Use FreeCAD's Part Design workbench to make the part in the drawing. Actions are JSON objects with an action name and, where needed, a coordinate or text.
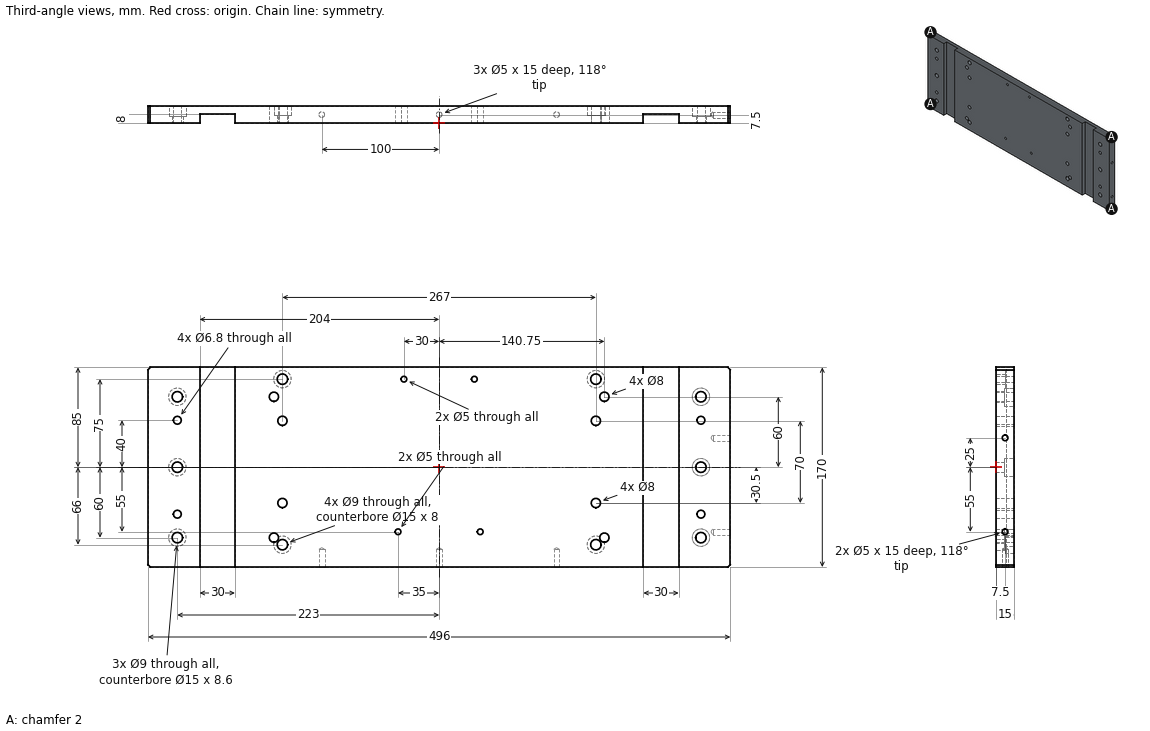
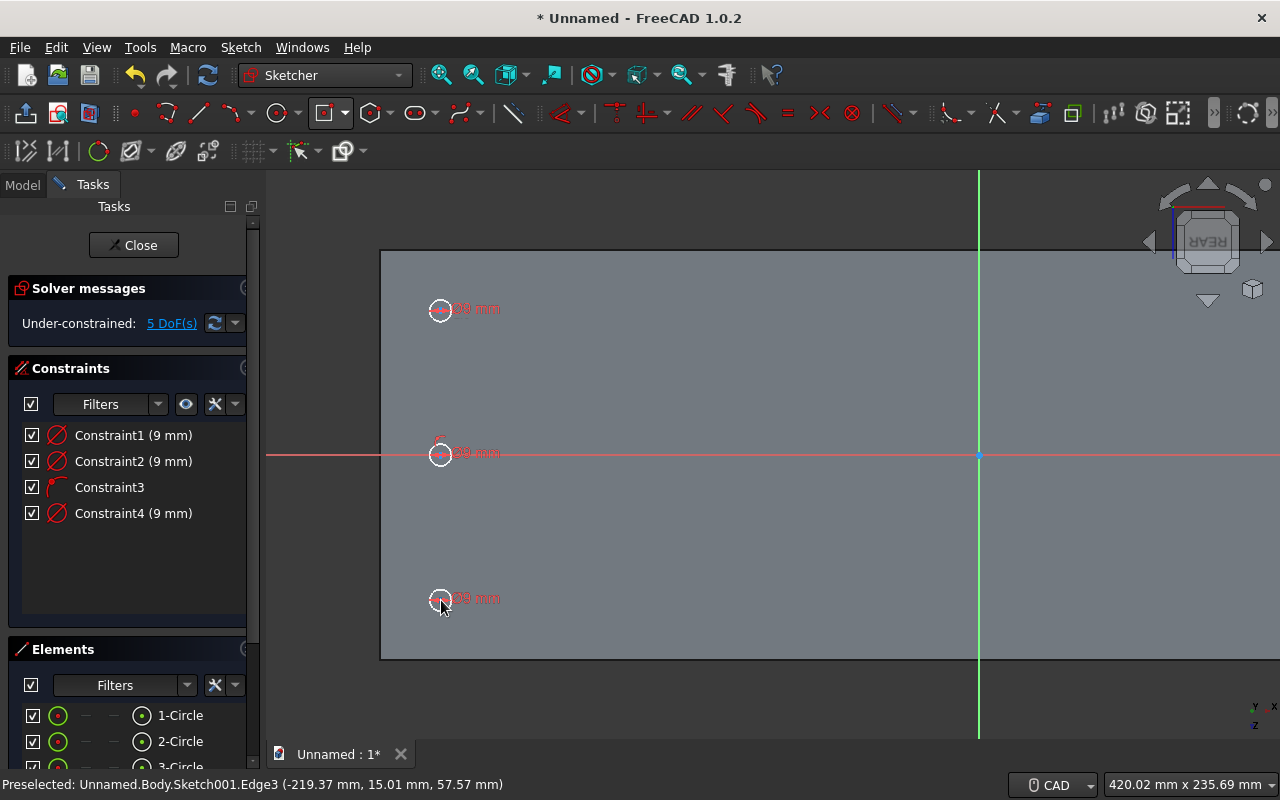
{"action": "left_click", "coordinate": [441, 311]}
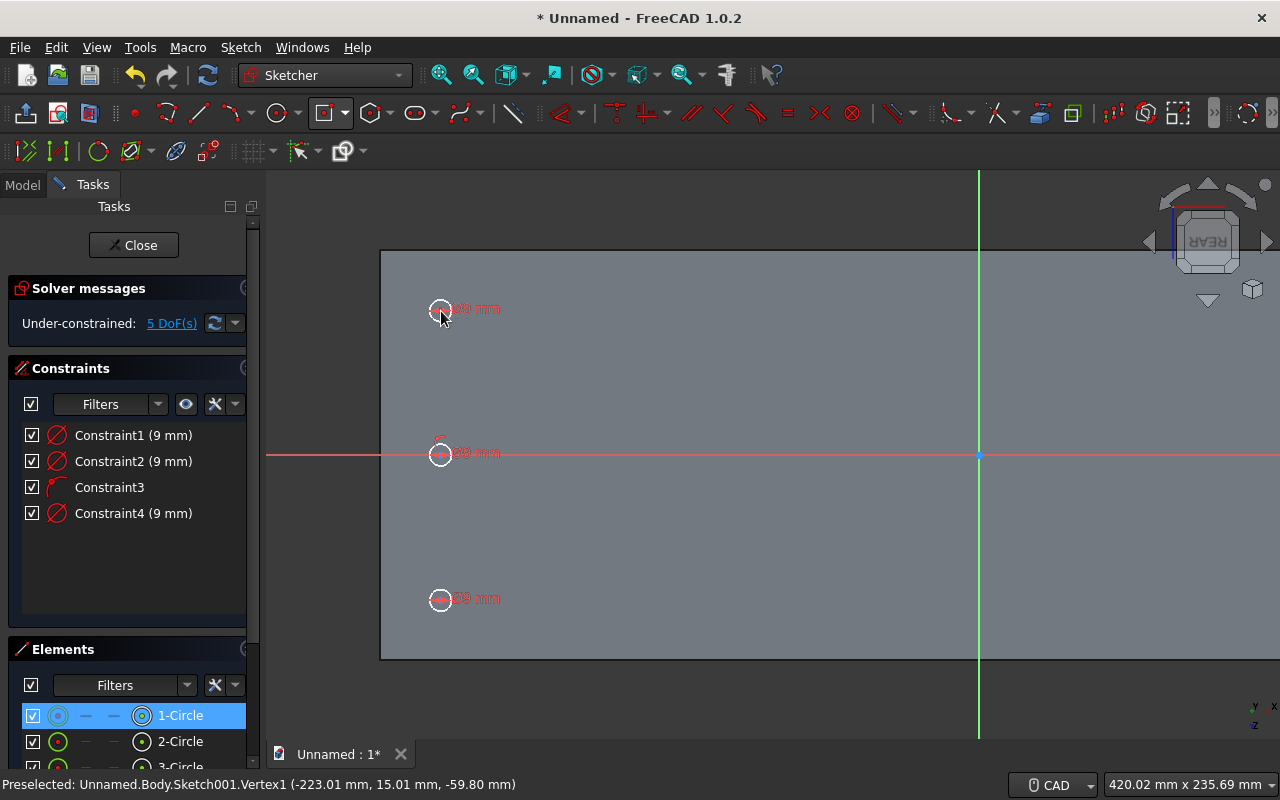
{"action": "left_click", "coordinate": [441, 600]}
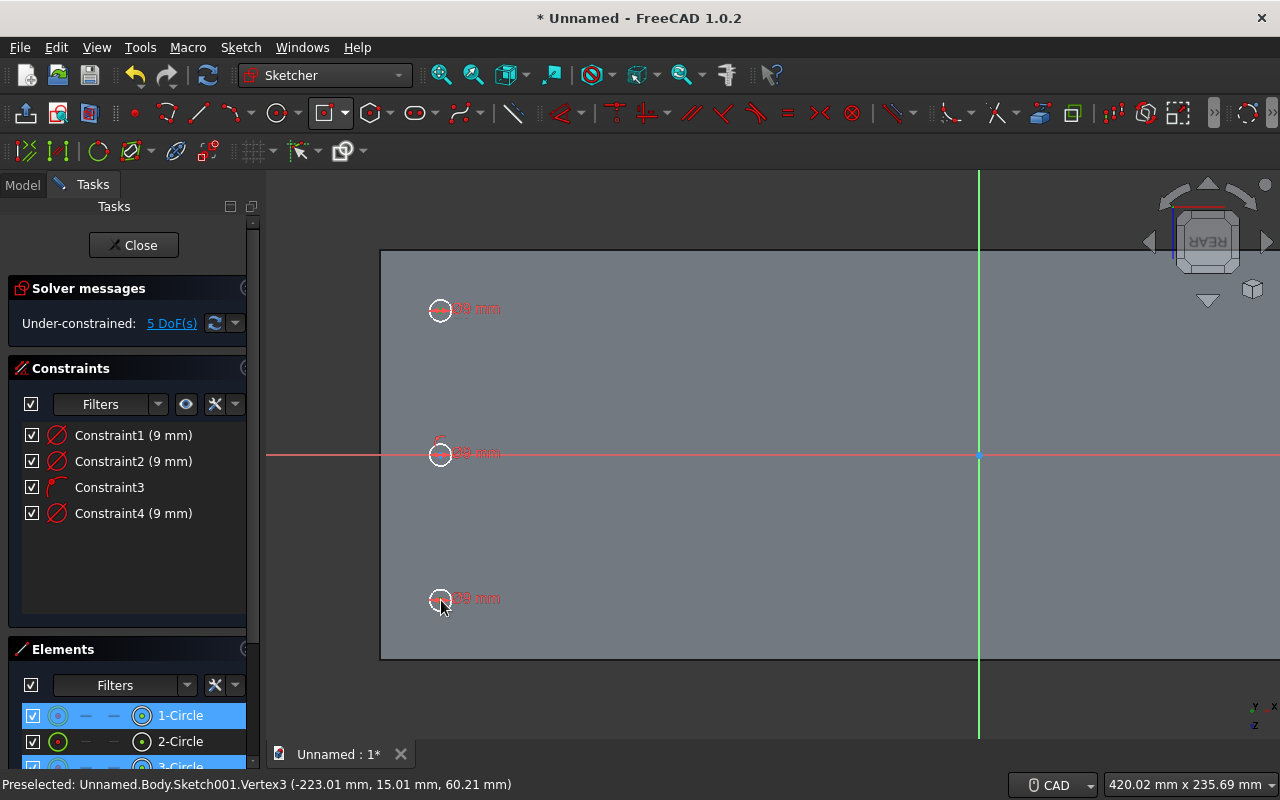
{"action": "left_click", "coordinate": [353, 455]}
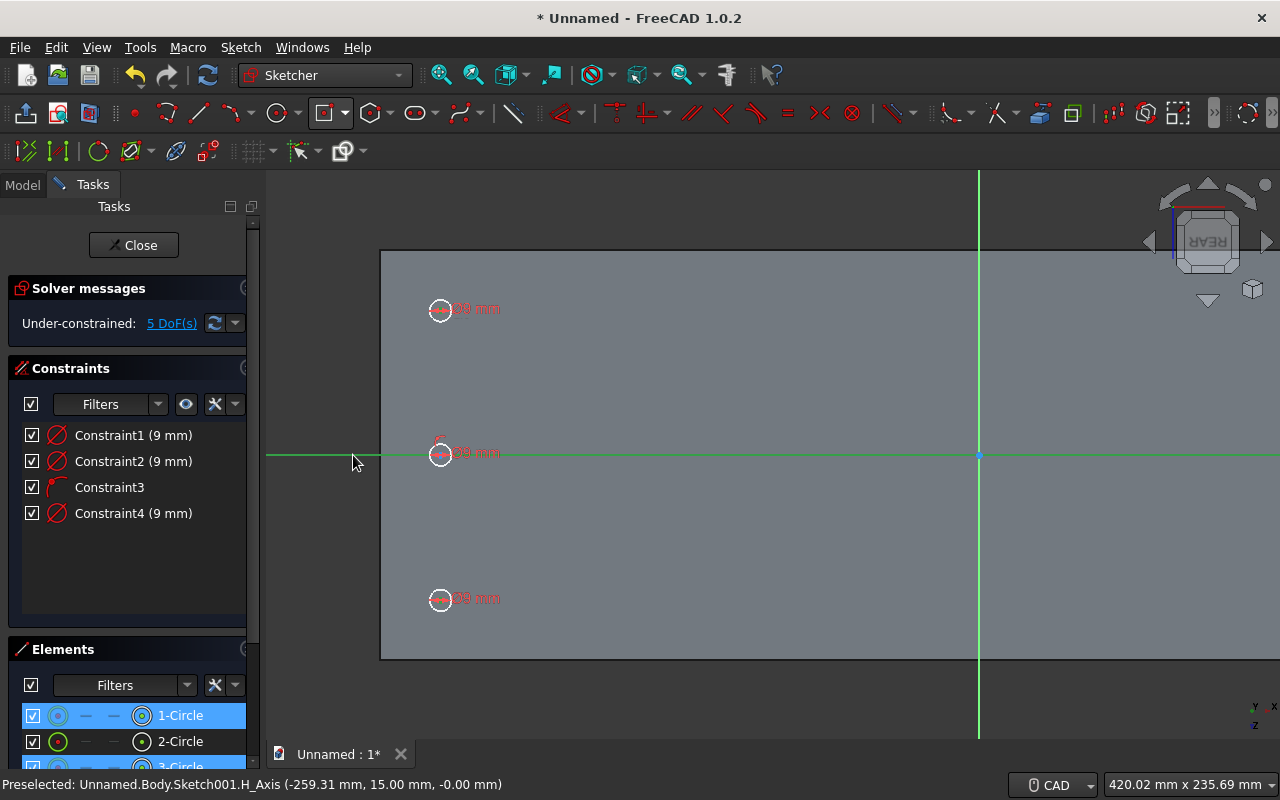
{"action": "left_click", "coordinate": [820, 114]}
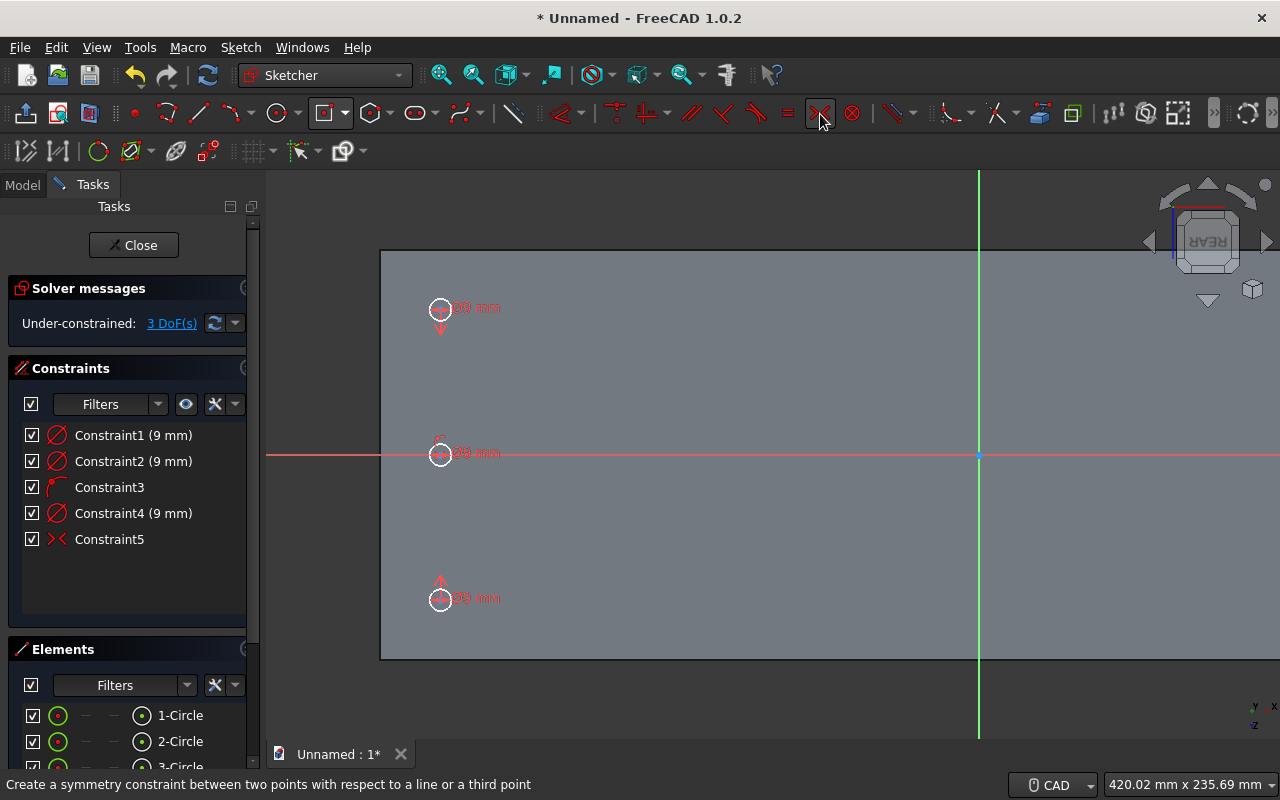
{"action": "left_click", "coordinate": [560, 114]}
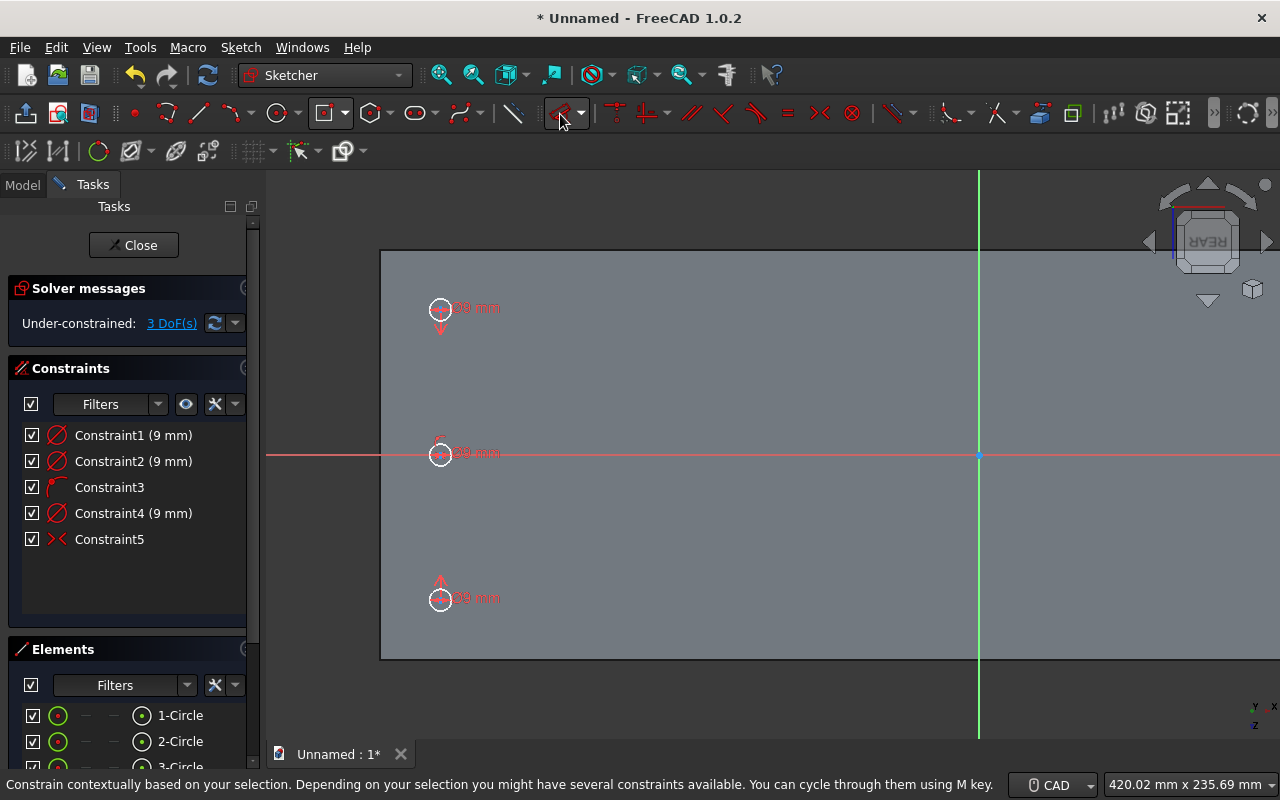
{"action": "left_click", "coordinate": [441, 310]}
{"action": "left_click", "coordinate": [1013, 382]}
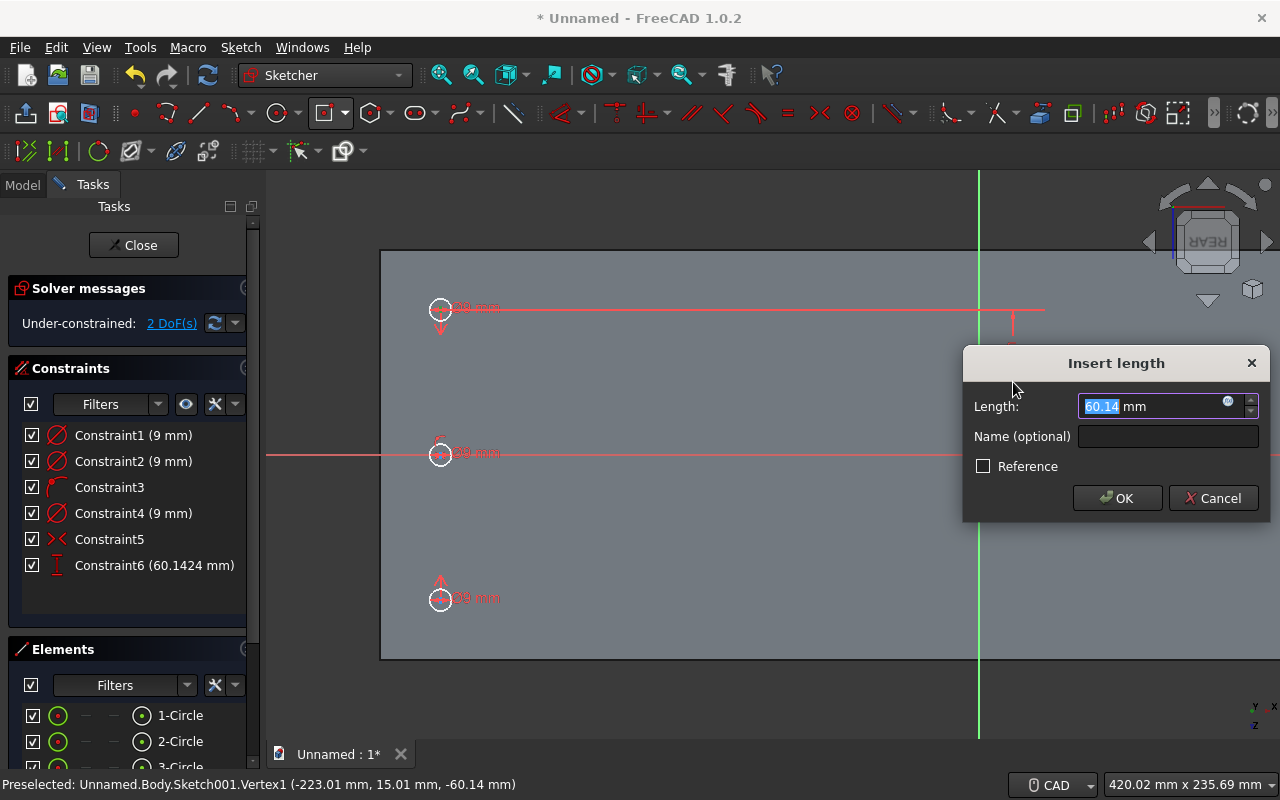
{"action": "type", "text": "60"}
{"action": "key", "text": "Return"}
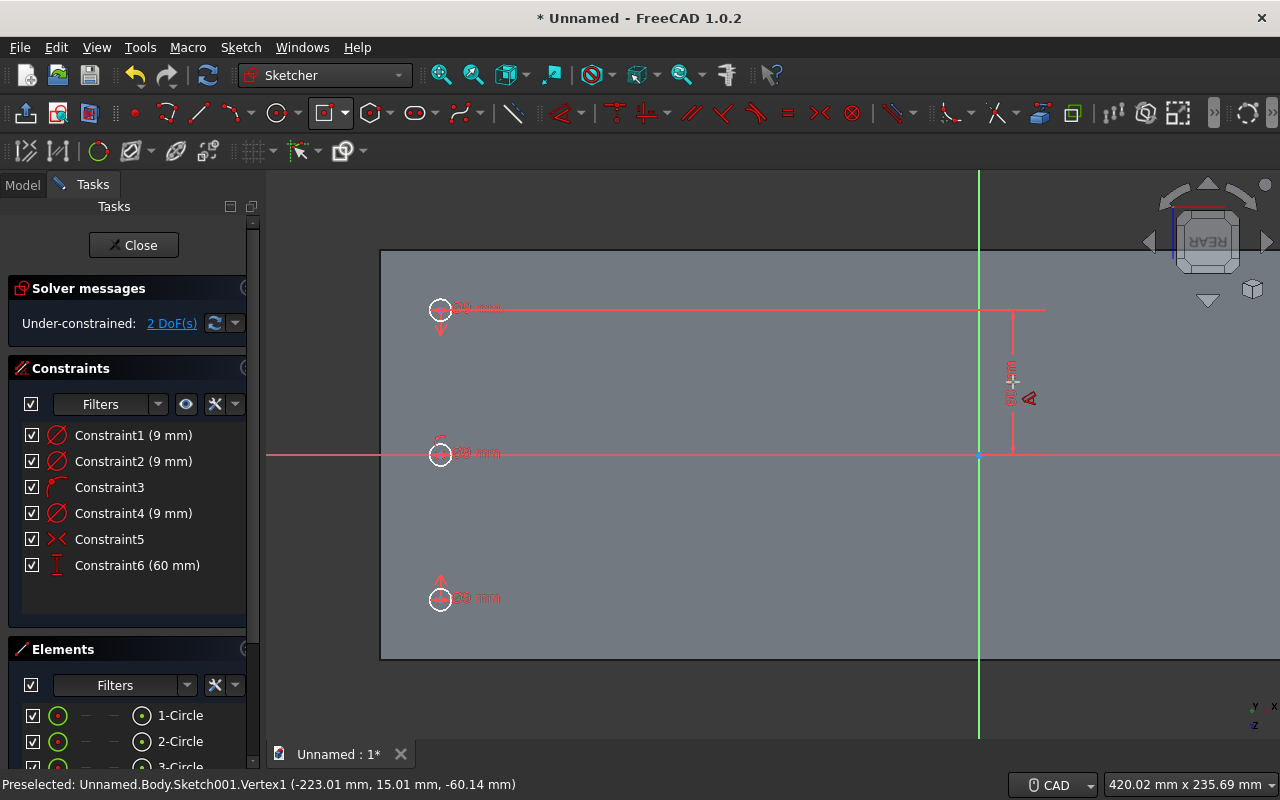
{"action": "left_click", "coordinate": [441, 310]}
{"action": "left_click", "coordinate": [710, 276]}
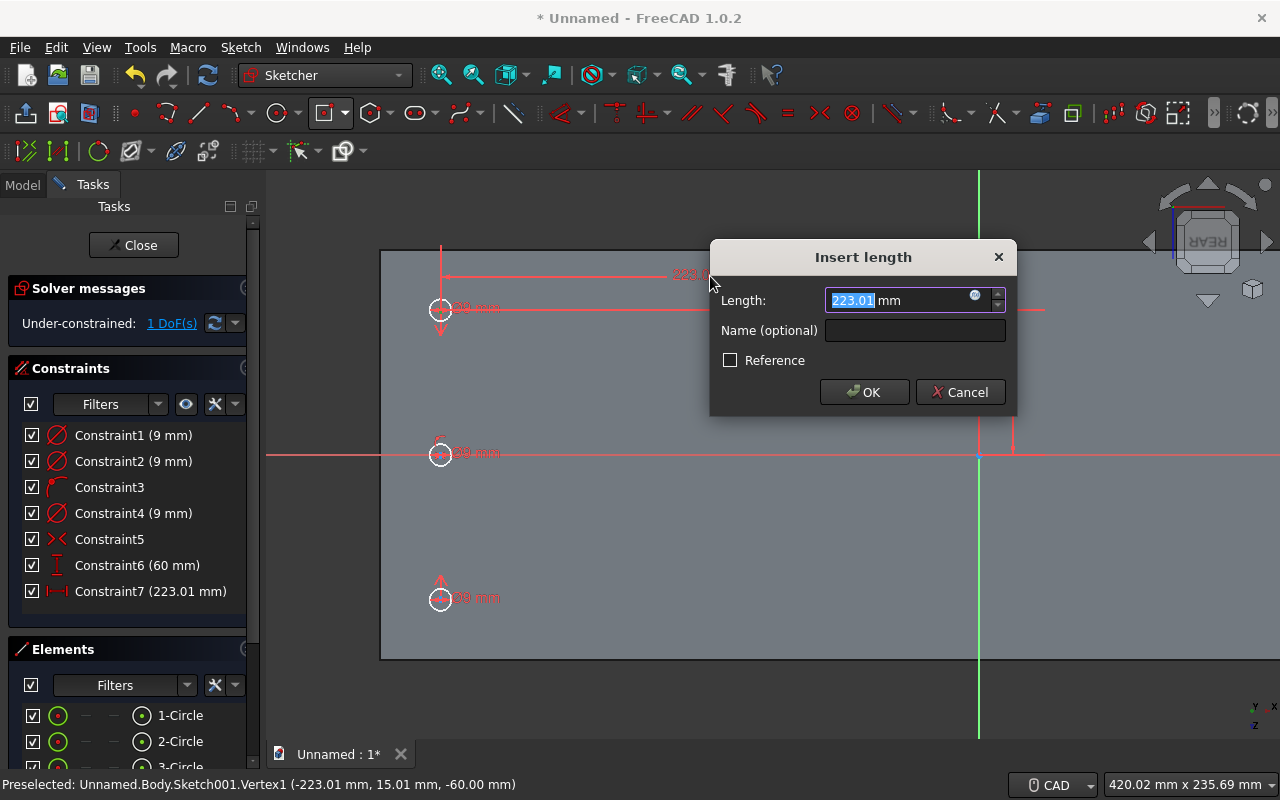
{"action": "type", "text": "223"}
{"action": "key", "text": "Return"}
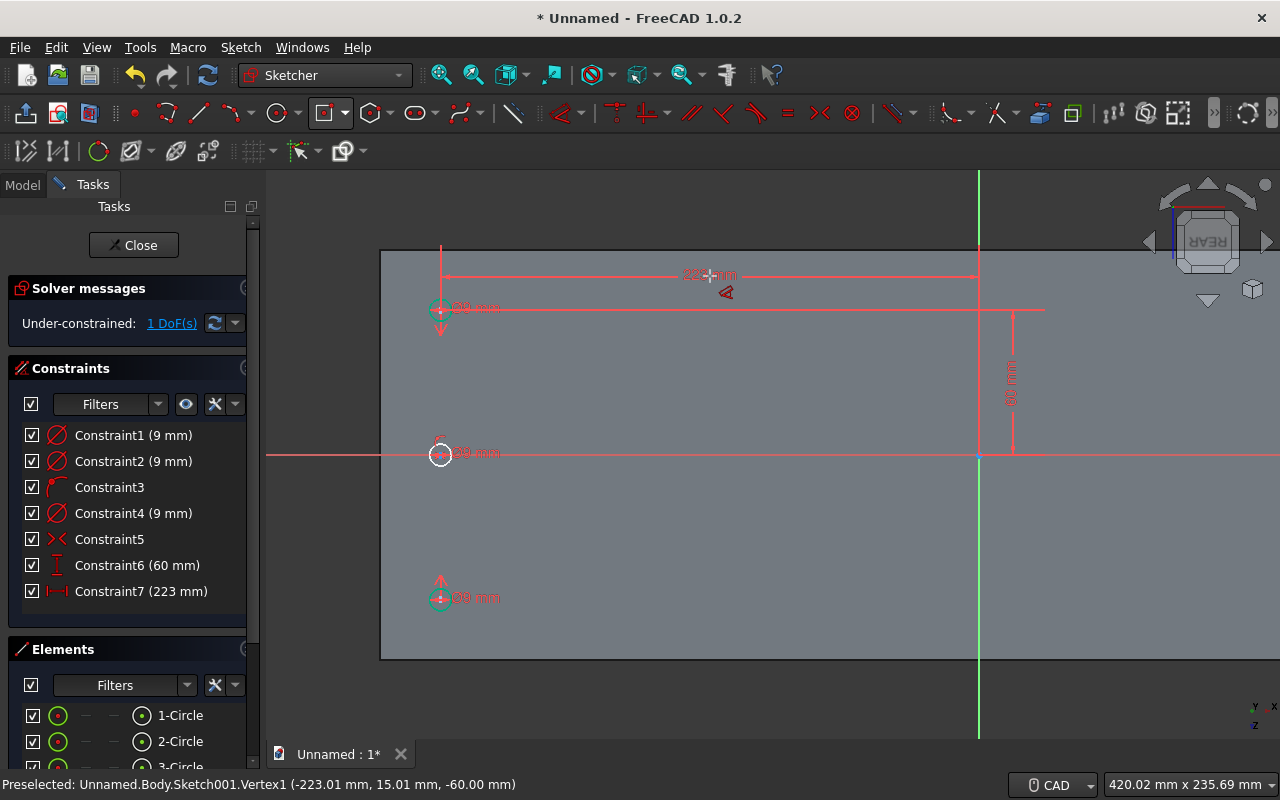
{"action": "left_click", "coordinate": [441, 455]}
{"action": "left_click", "coordinate": [710, 489]}